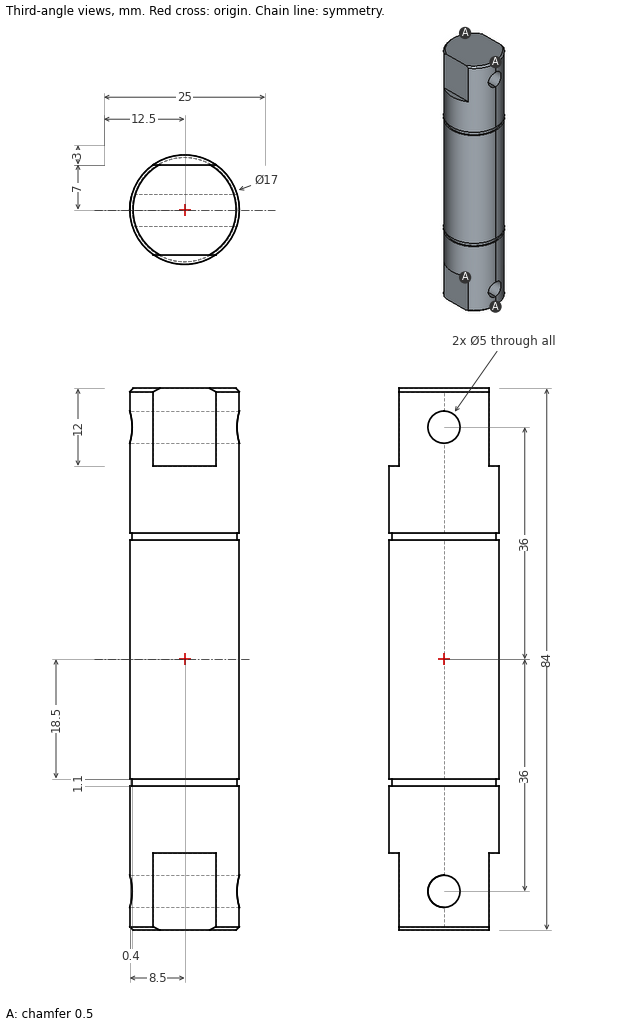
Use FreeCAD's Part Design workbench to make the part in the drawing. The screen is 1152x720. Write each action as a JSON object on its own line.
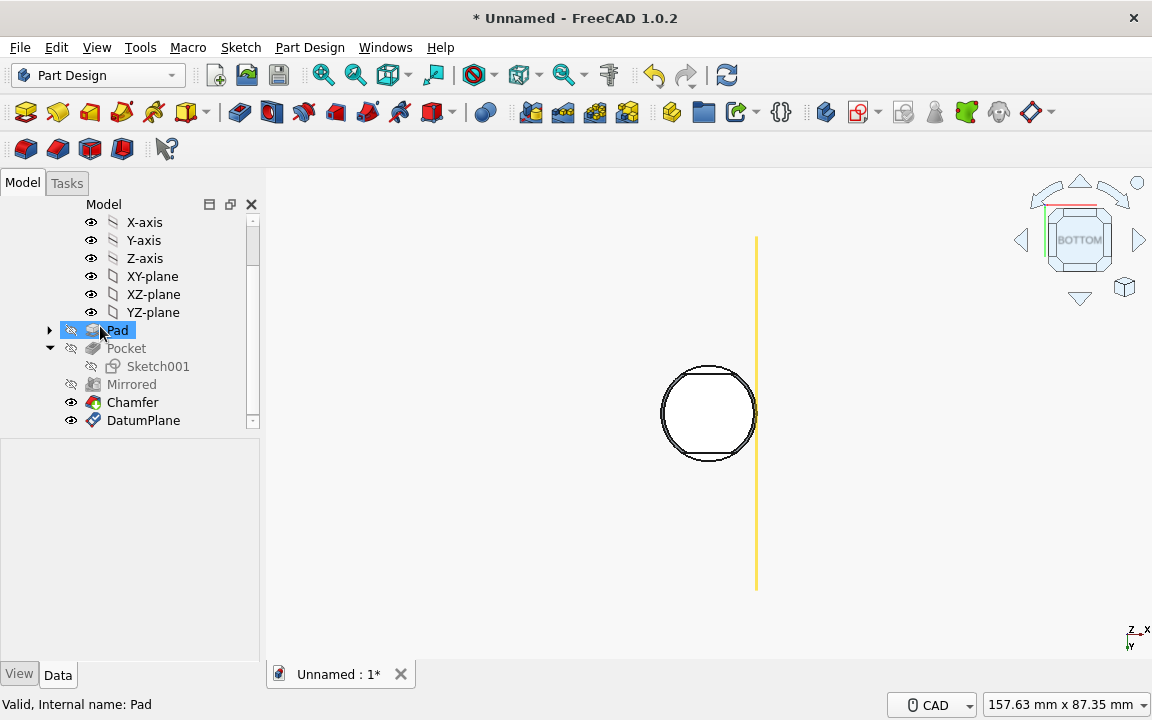
{"action": "left_click", "coordinate": [116, 420]}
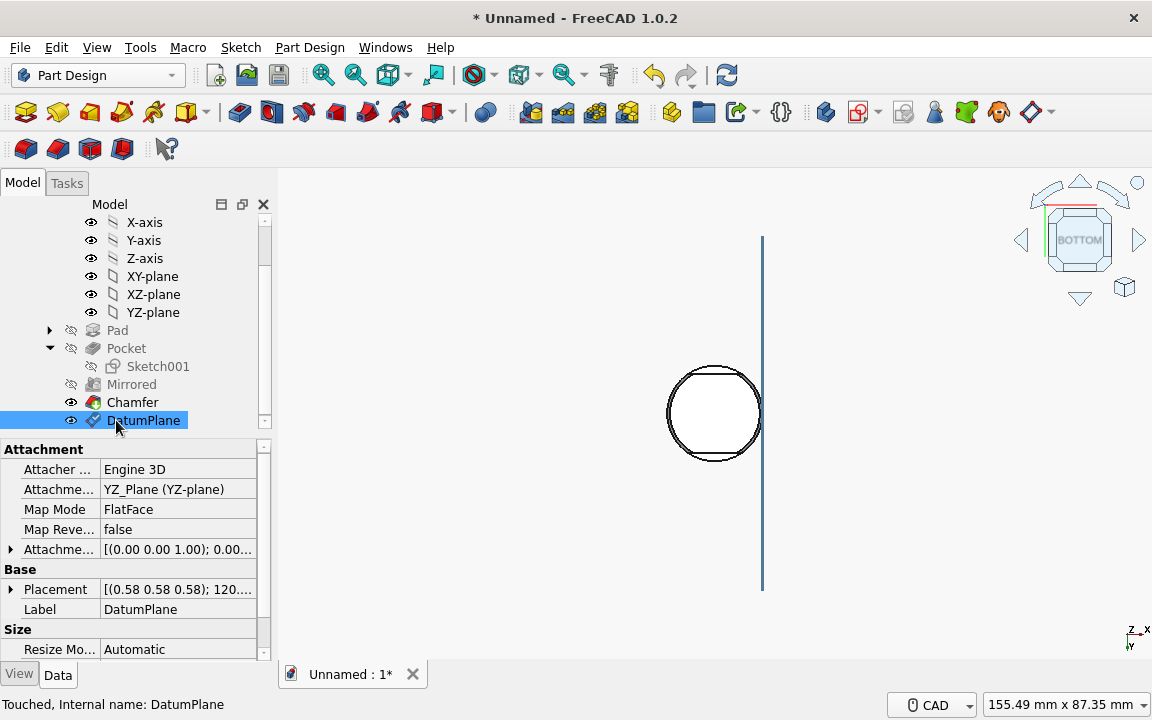
{"action": "left_click", "coordinate": [858, 112]}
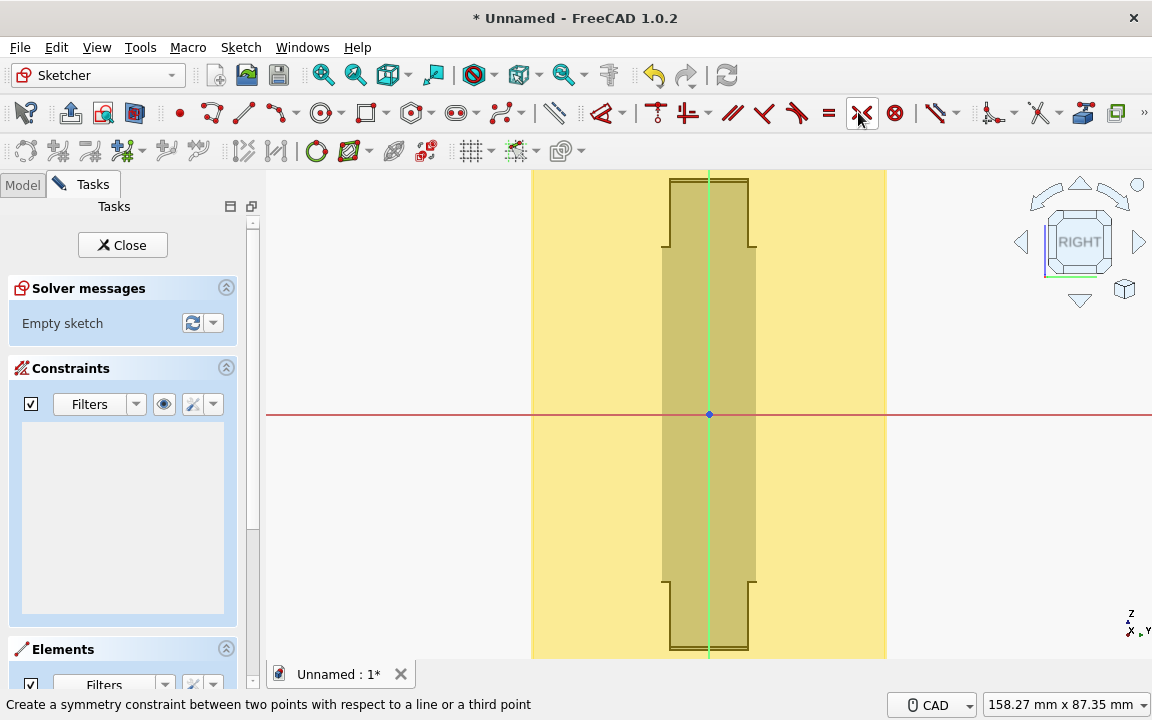
{"action": "scroll", "coordinate": [501, 414], "scroll_direction": "down", "scroll_amount": 2}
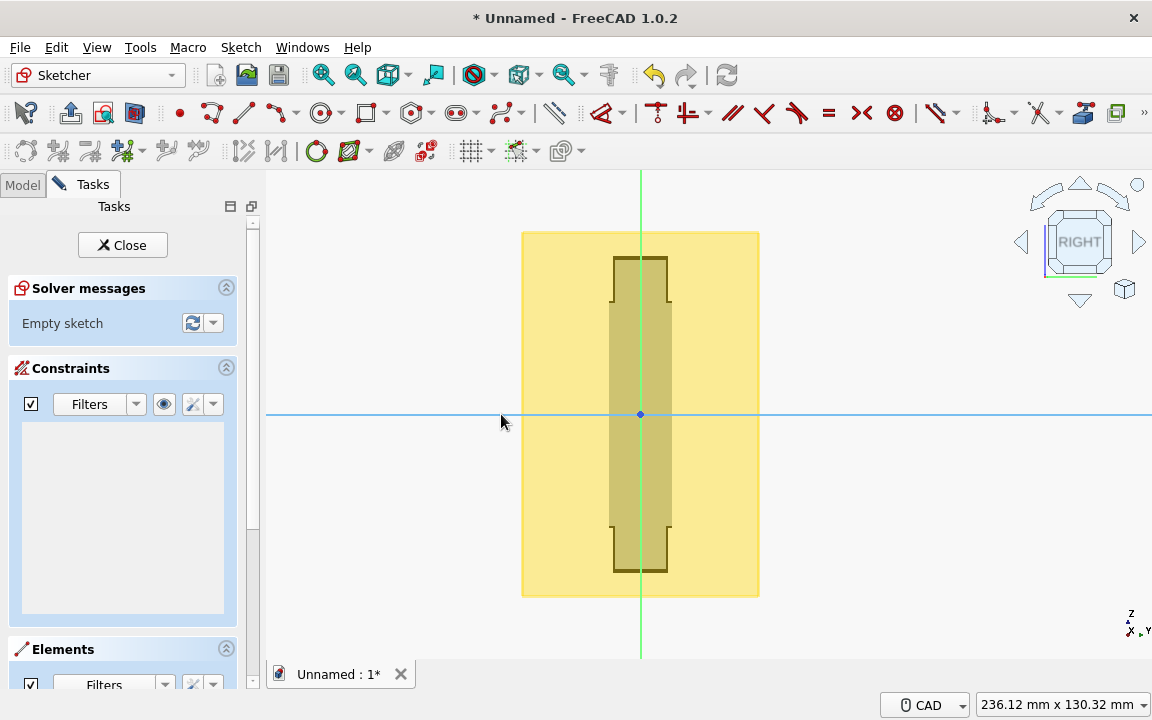
{"action": "left_click", "coordinate": [322, 114]}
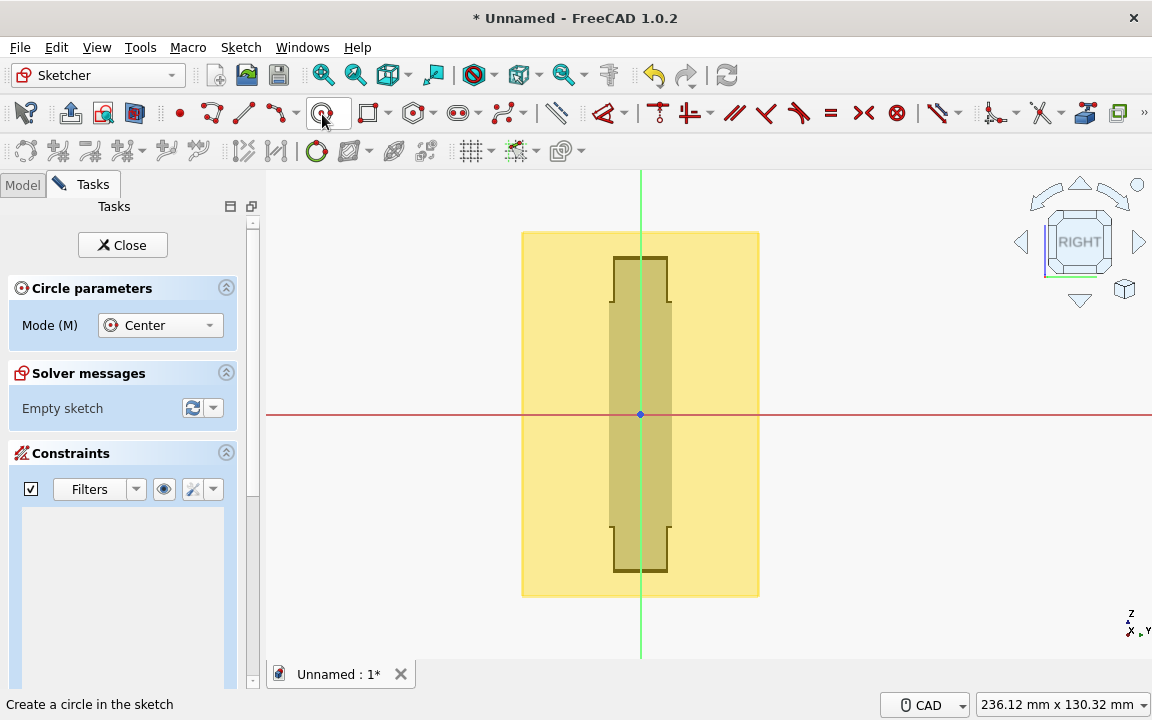
{"action": "scroll", "coordinate": [641, 279], "scroll_direction": "up", "scroll_amount": 5}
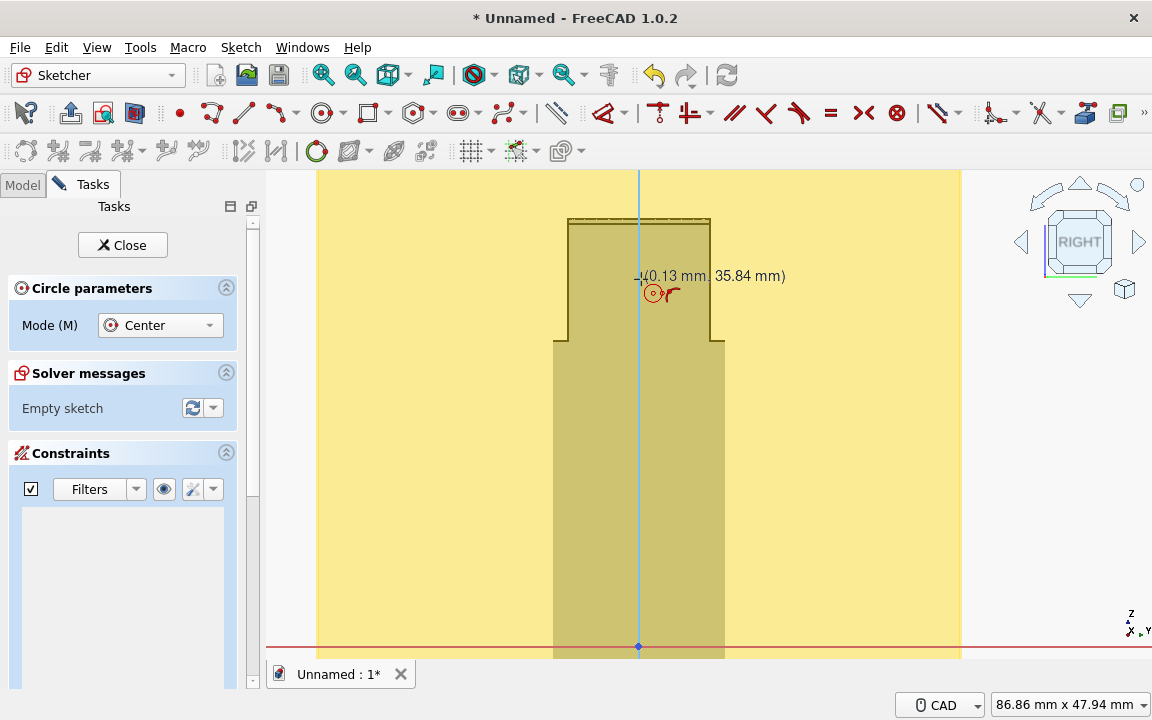
{"action": "left_click", "coordinate": [639, 280]}
{"action": "left_click", "coordinate": [657, 262]}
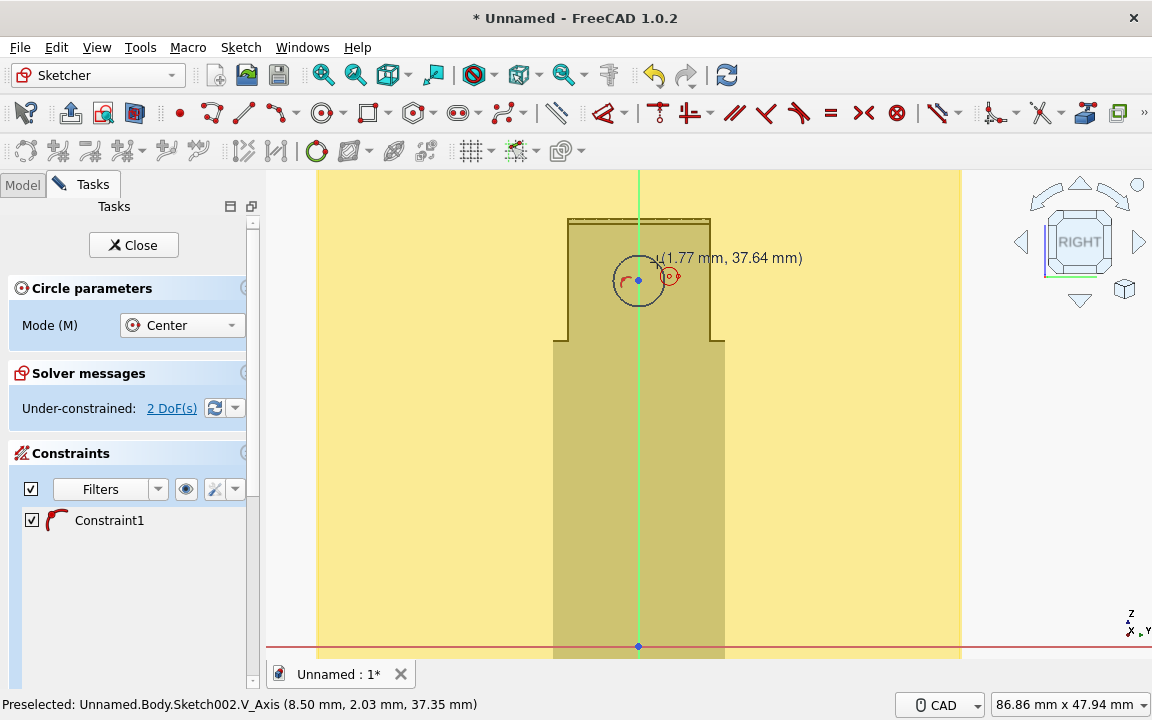
{"action": "scroll", "coordinate": [641, 279], "scroll_direction": "down", "scroll_amount": 5}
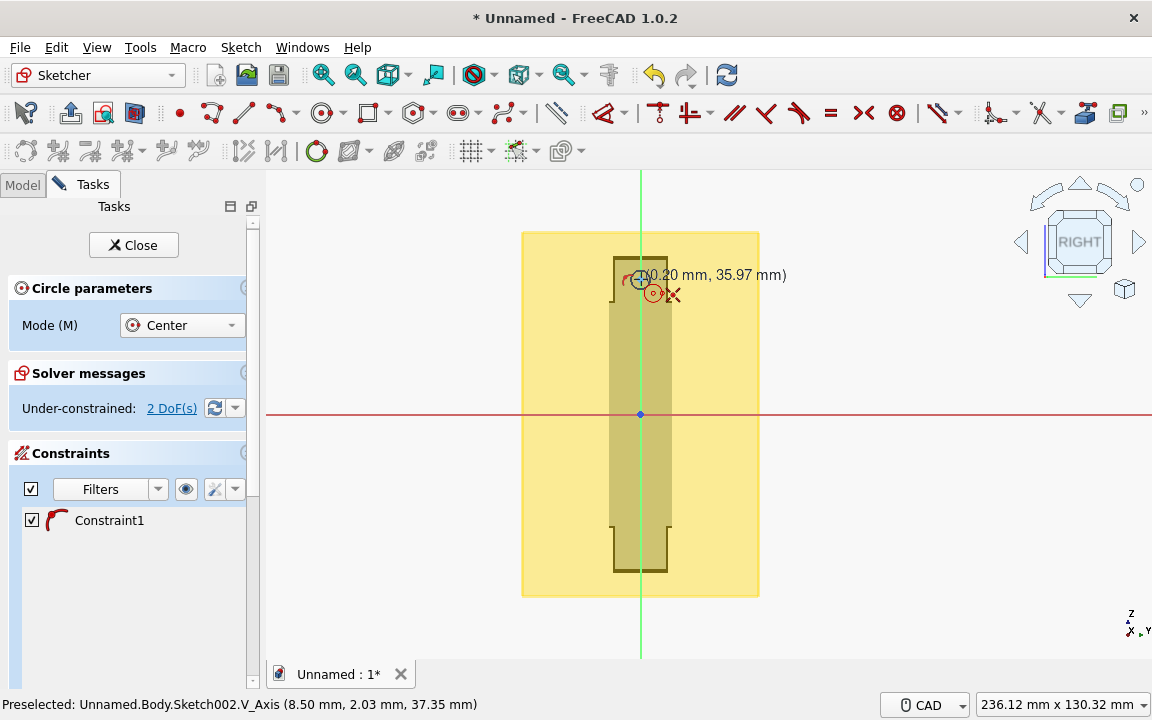
{"action": "scroll", "coordinate": [641, 550], "scroll_direction": "up", "scroll_amount": 5}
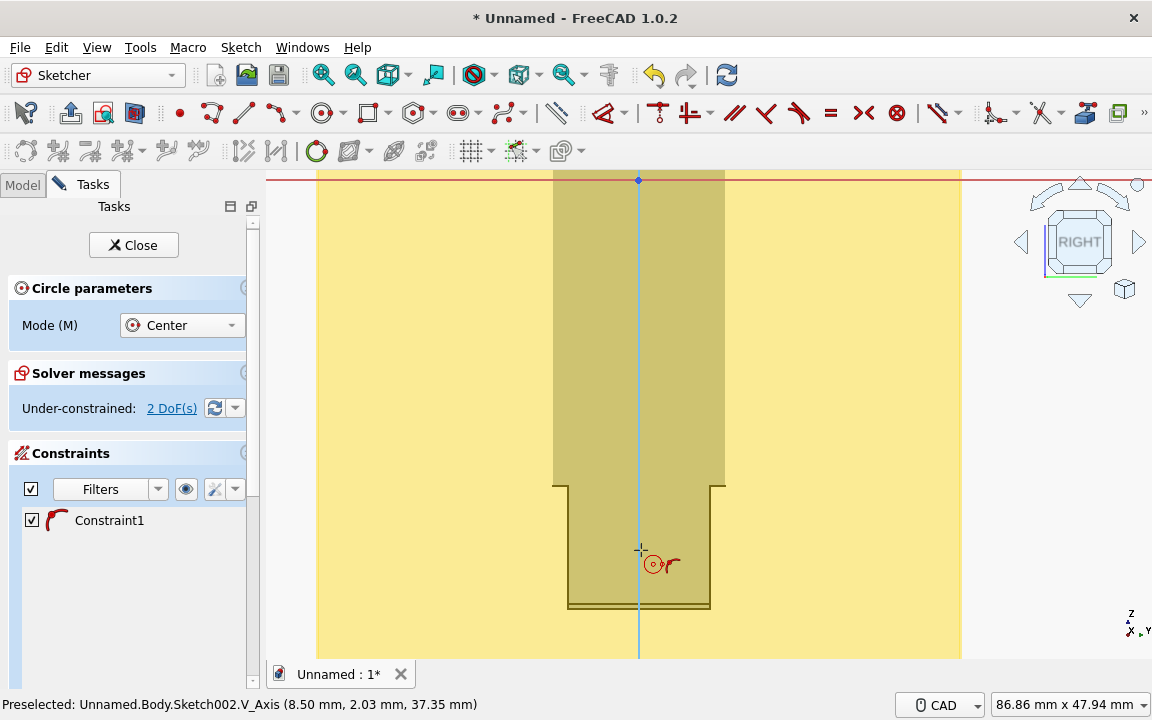
{"action": "left_click", "coordinate": [639, 548]}
{"action": "left_click", "coordinate": [657, 530]}
{"action": "key", "text": "Escape"}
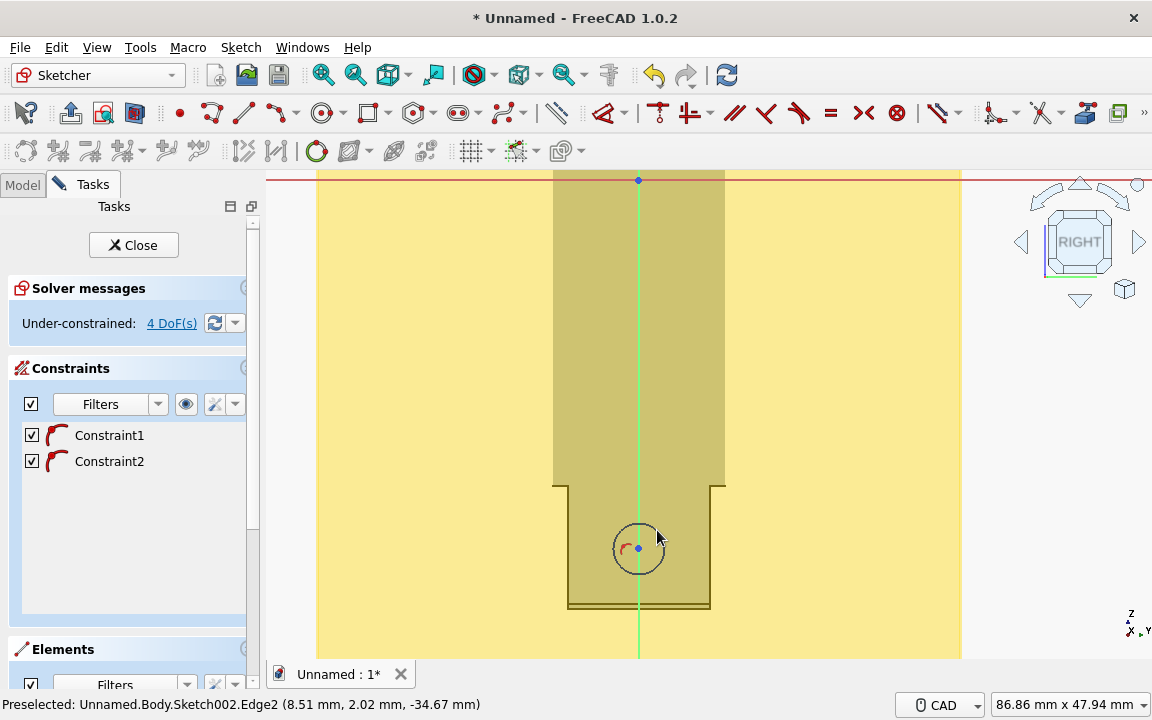
{"action": "scroll", "coordinate": [641, 551], "scroll_direction": "down", "scroll_amount": 5}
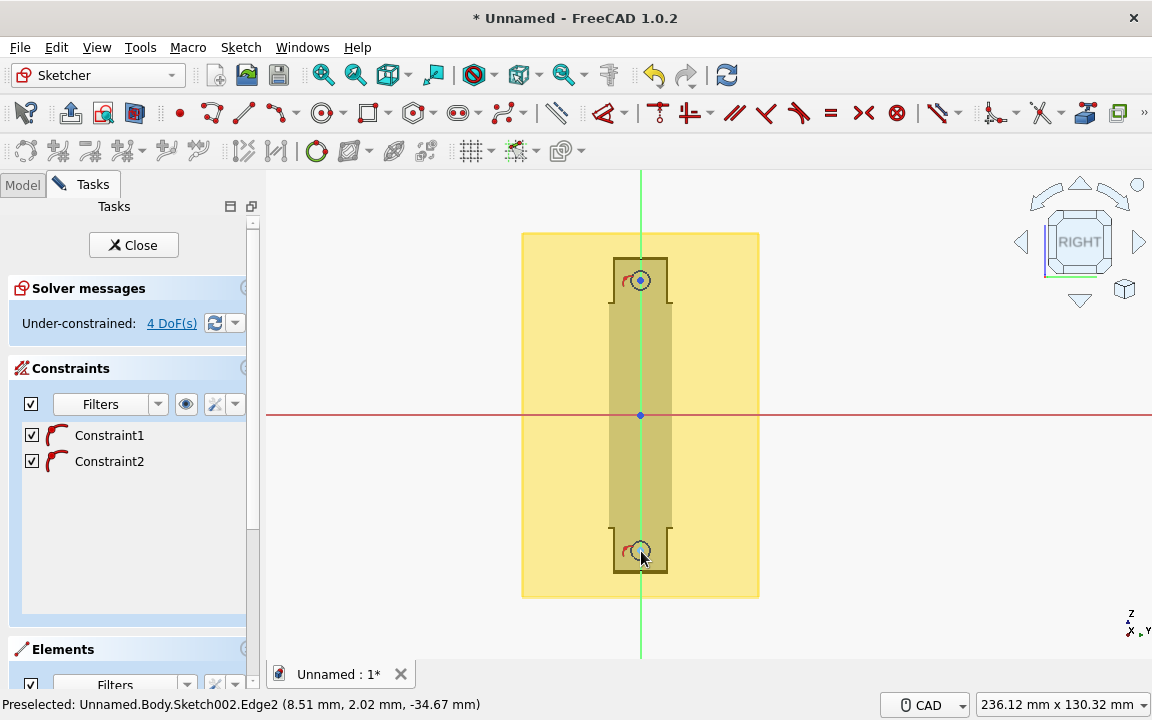
{"action": "scroll", "coordinate": [647, 274], "scroll_direction": "up", "scroll_amount": 4}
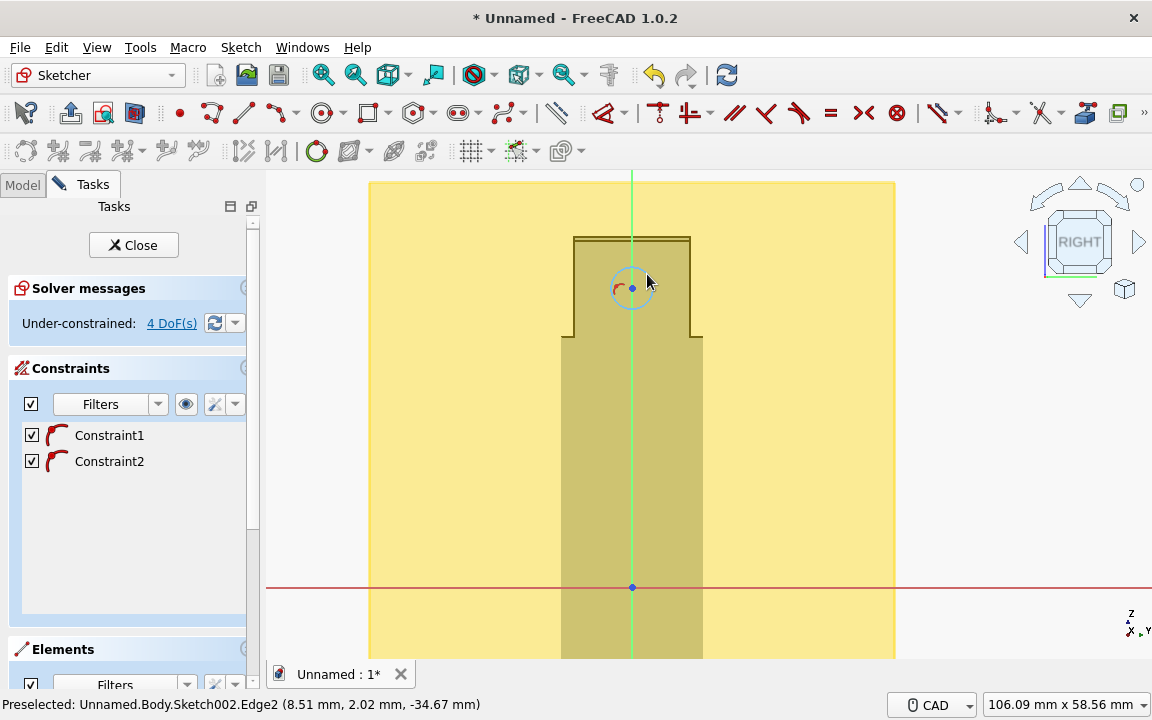
{"action": "left_click", "coordinate": [647, 273]}